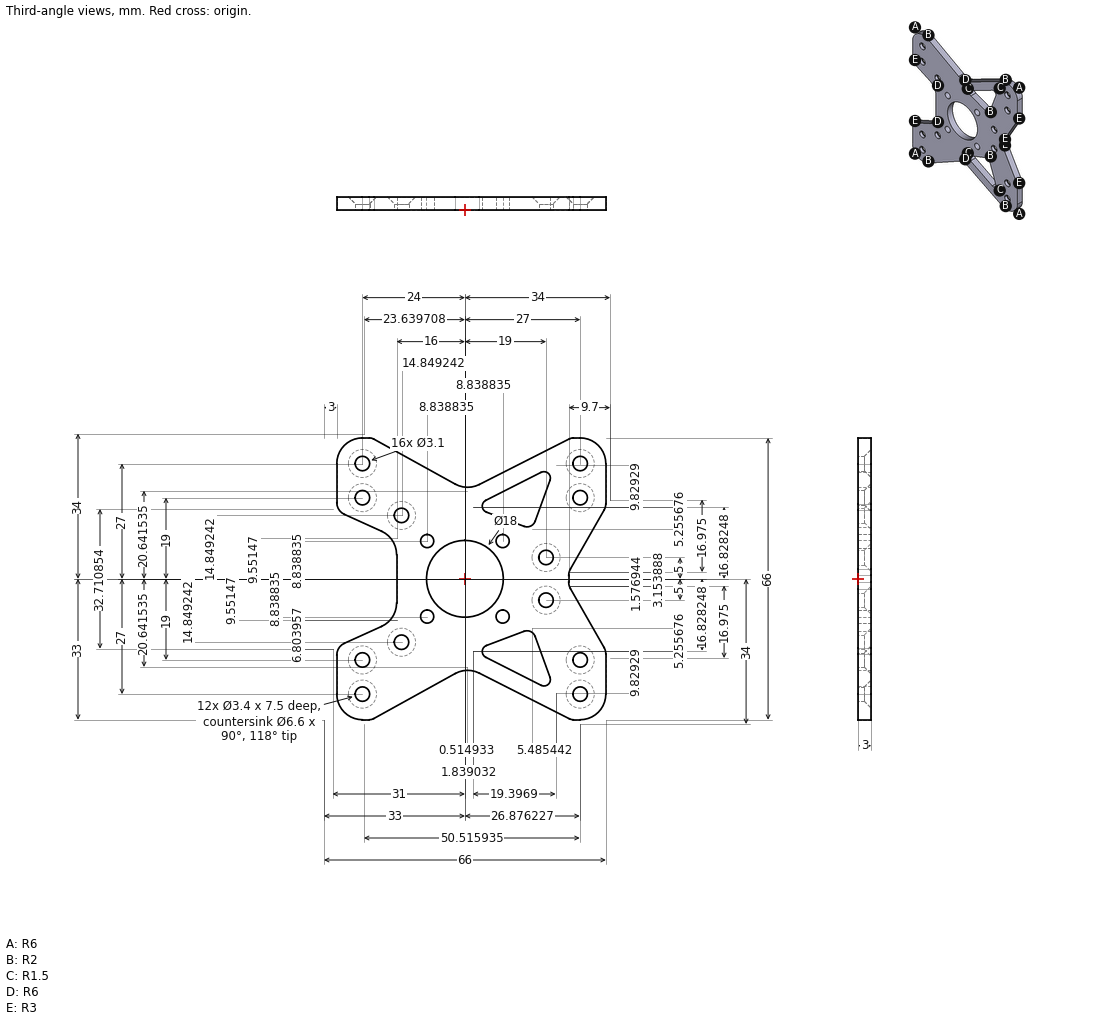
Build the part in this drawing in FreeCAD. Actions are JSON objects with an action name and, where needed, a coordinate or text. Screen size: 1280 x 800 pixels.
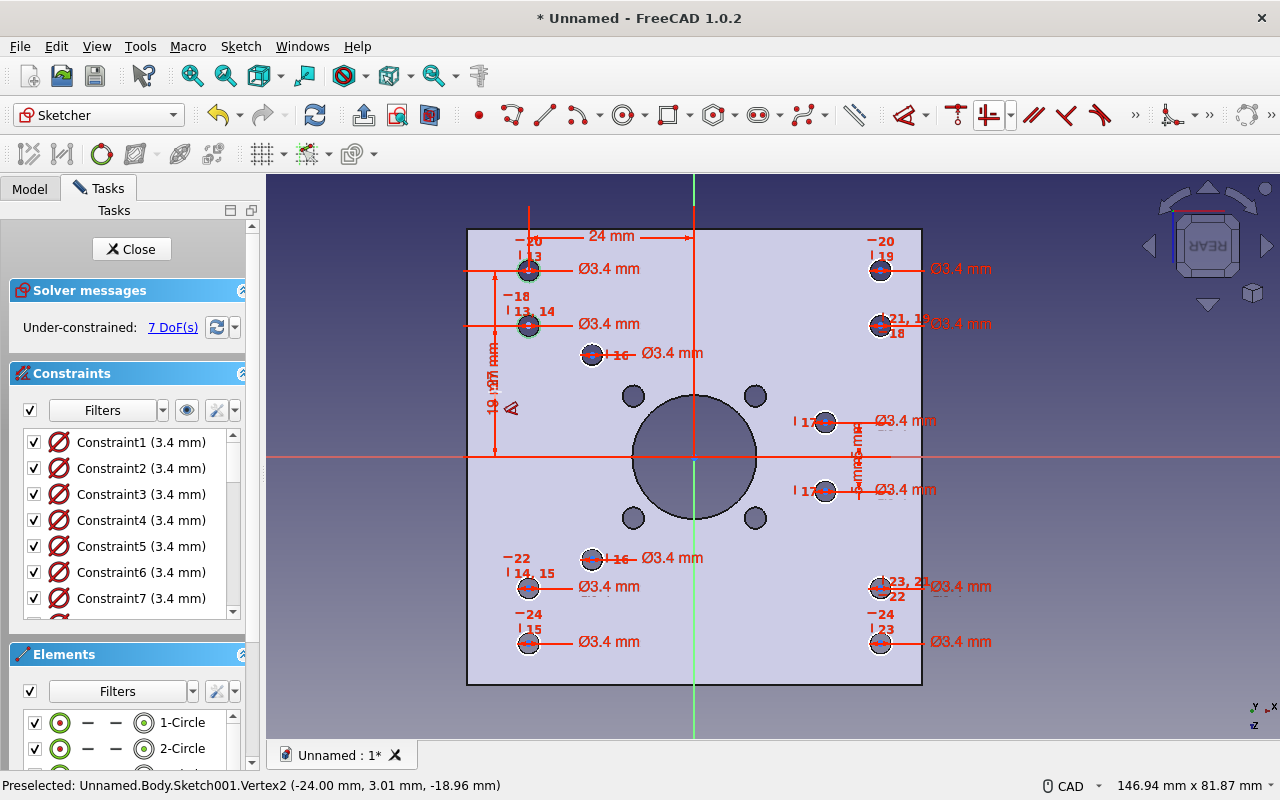
{"action": "left_click", "coordinate": [529, 589]}
{"action": "left_click", "coordinate": [495, 523]}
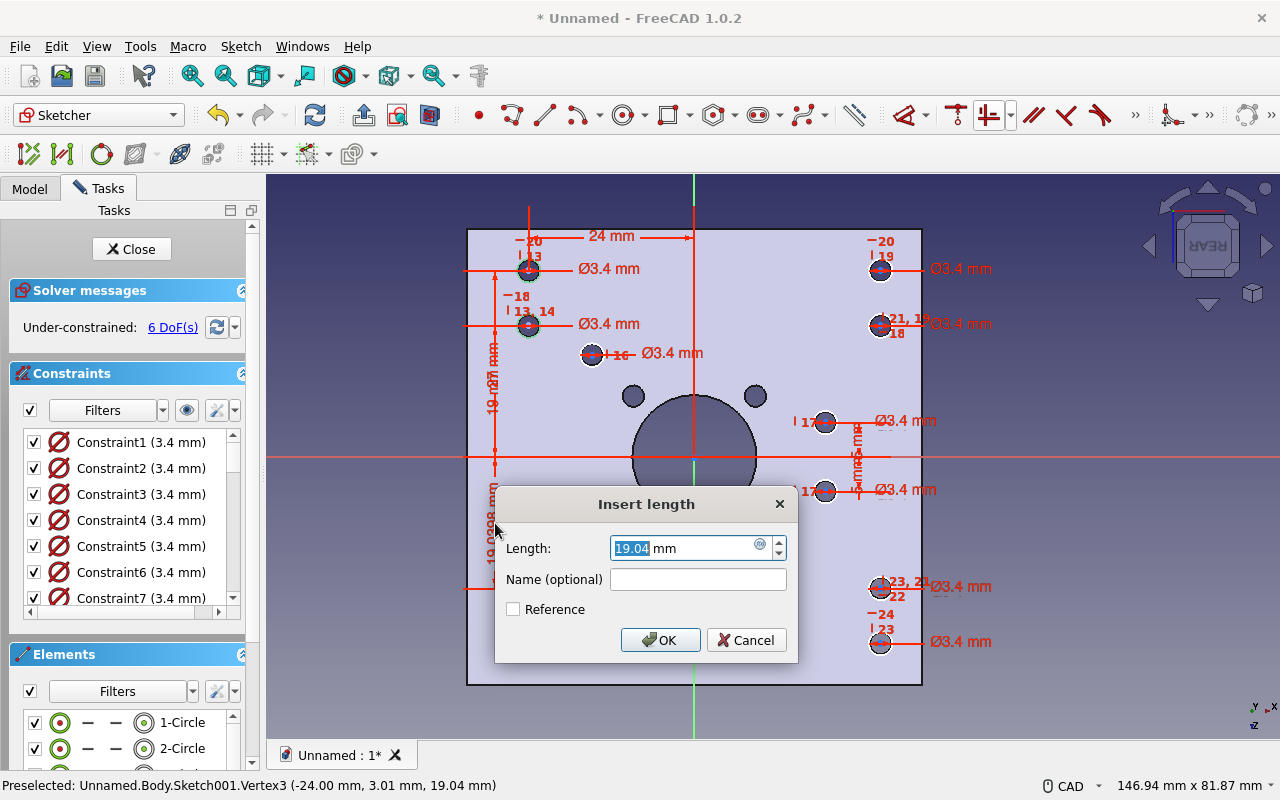
{"action": "type", "text": "19"}
{"action": "key", "text": "Return"}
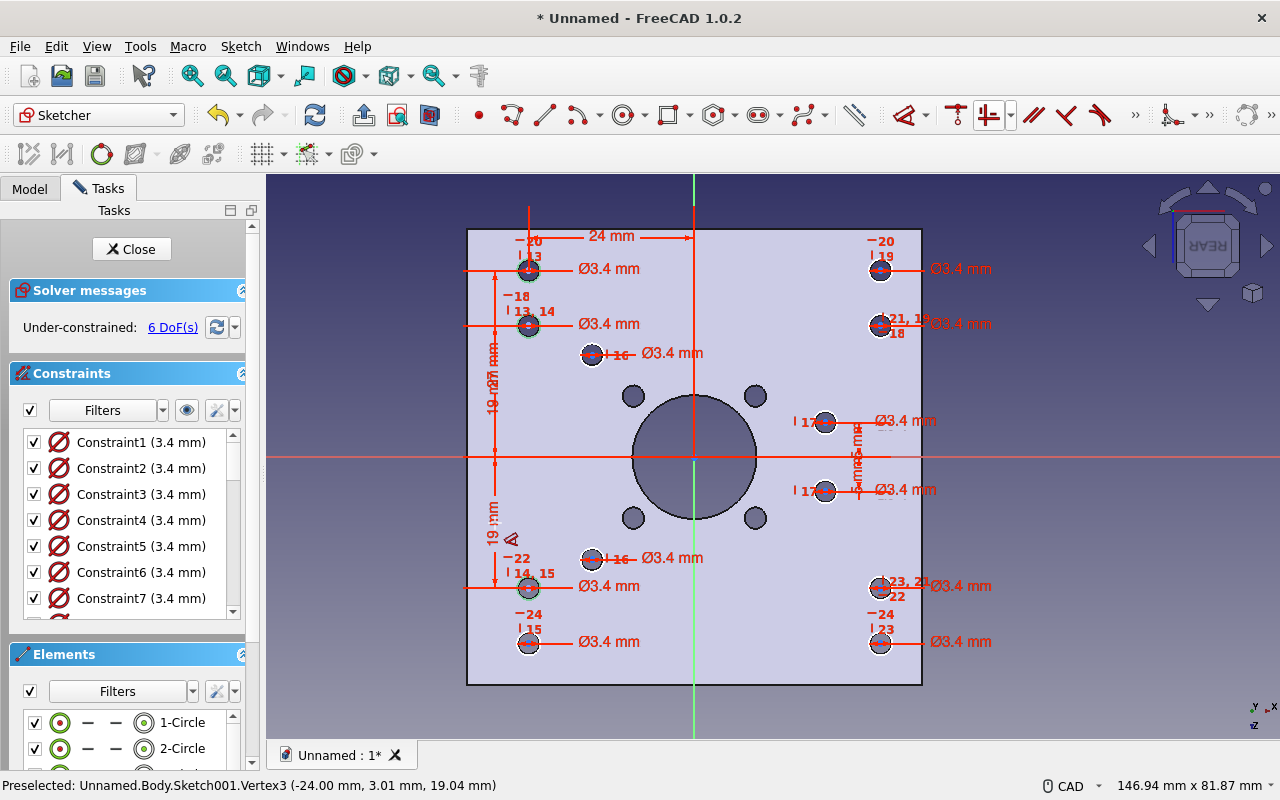
{"action": "left_click", "coordinate": [529, 644]}
{"action": "left_click", "coordinate": [495, 550]}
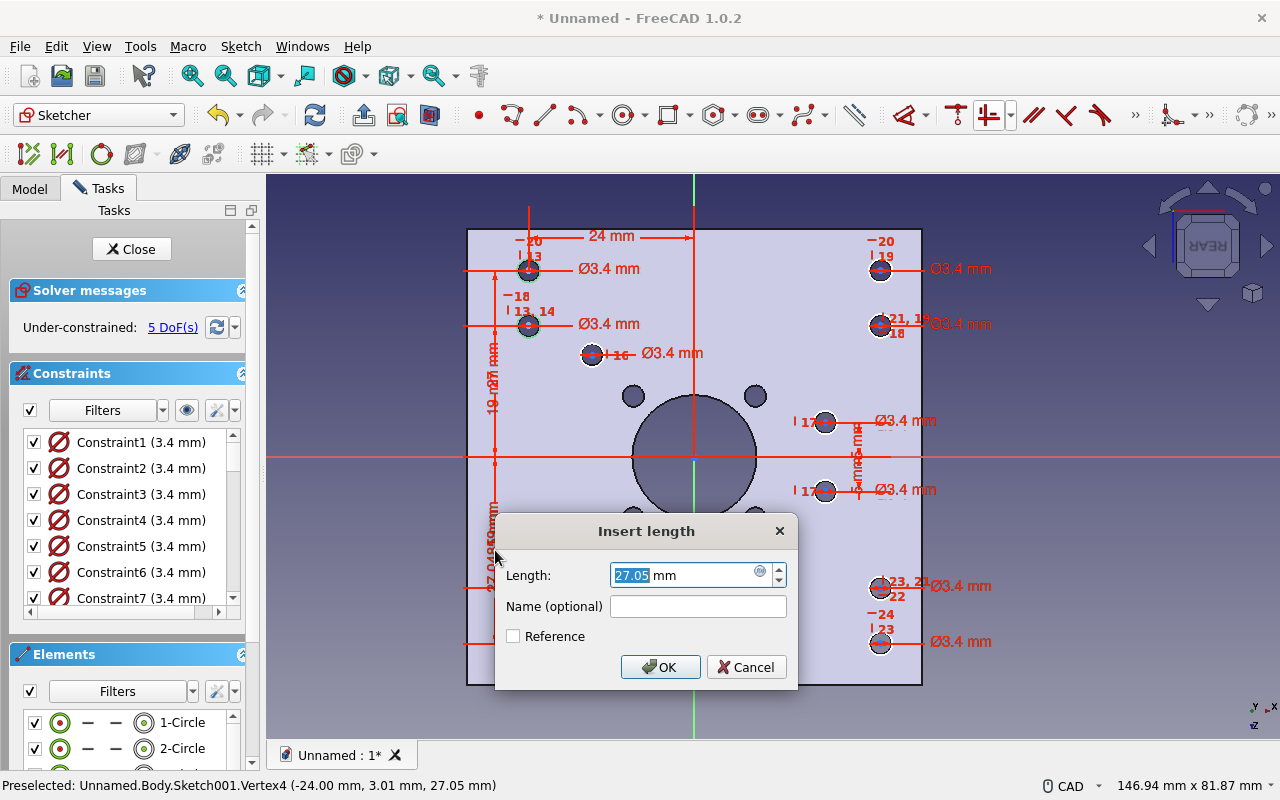
{"action": "type", "text": "27"}
{"action": "key", "text": "Return"}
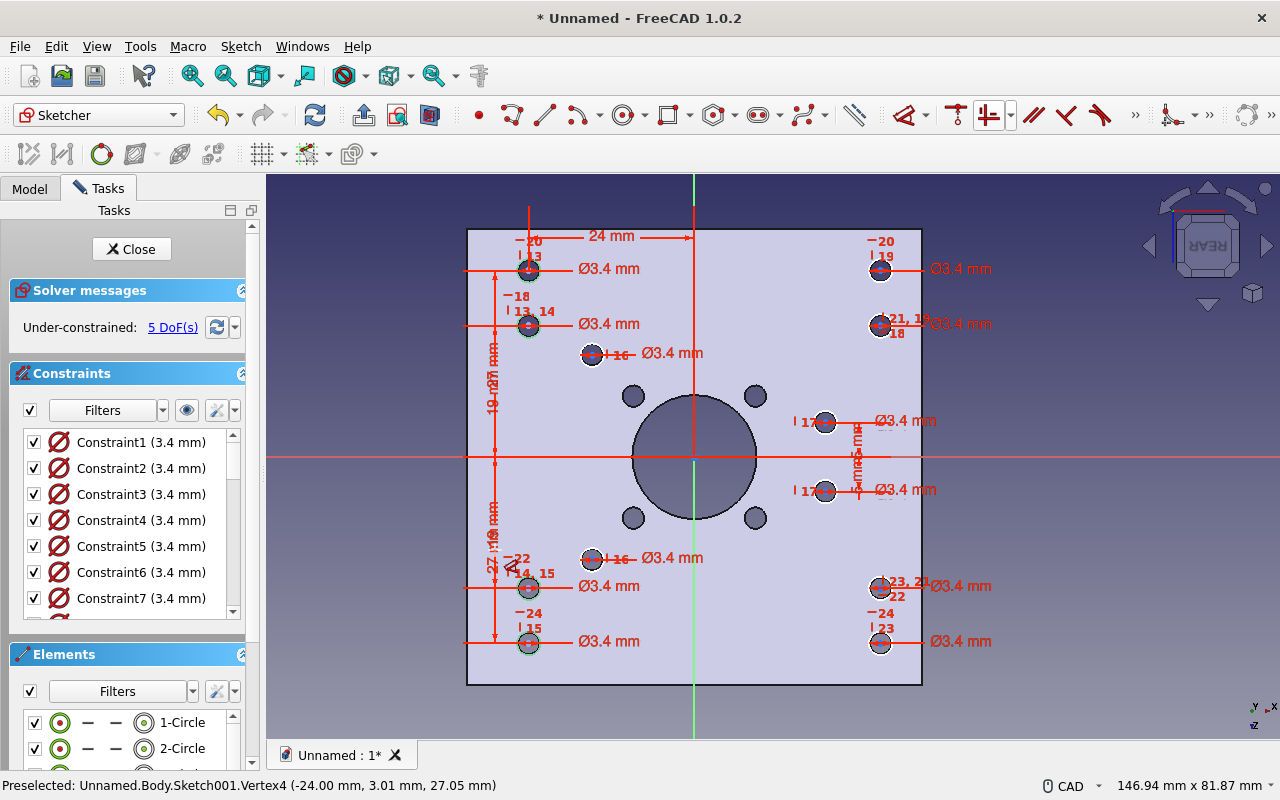
{"action": "left_click", "coordinate": [825, 492]}
{"action": "left_click", "coordinate": [760, 526]}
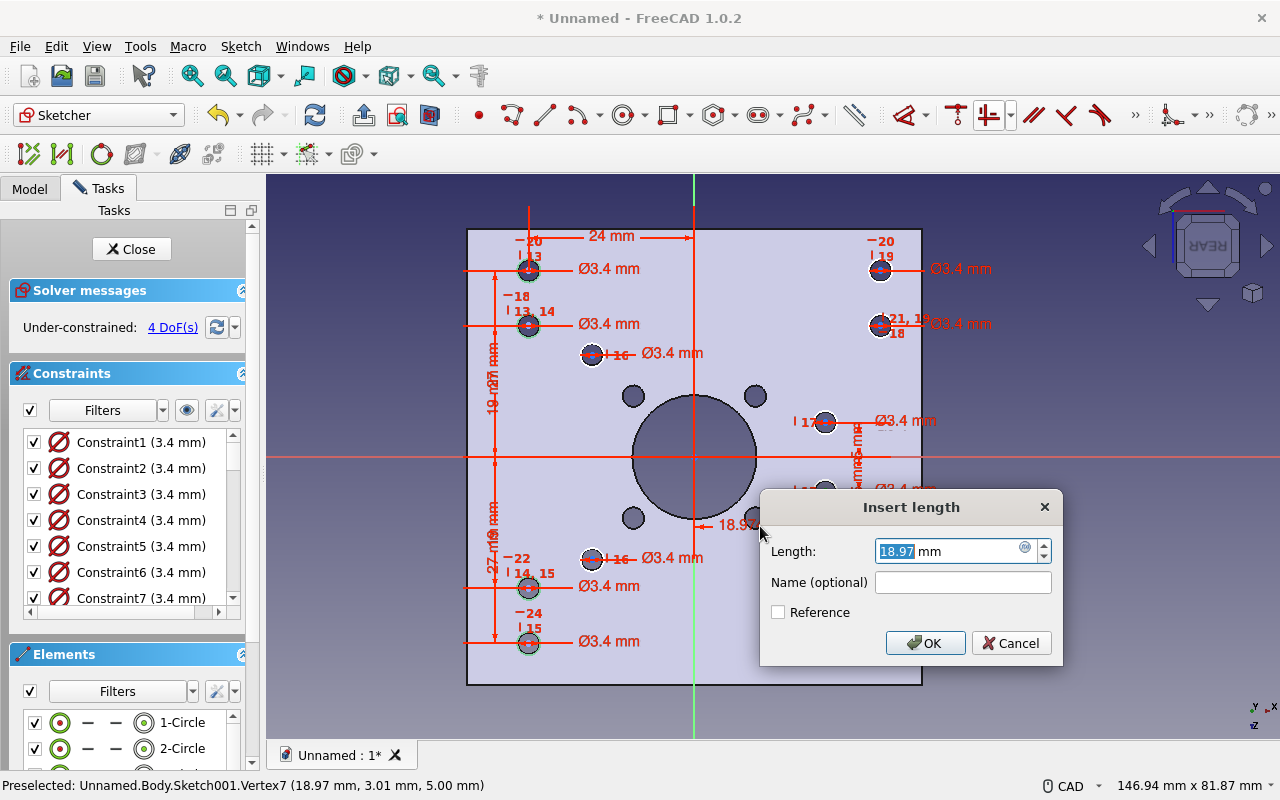
{"action": "type", "text": "19"}
{"action": "key", "text": "Return"}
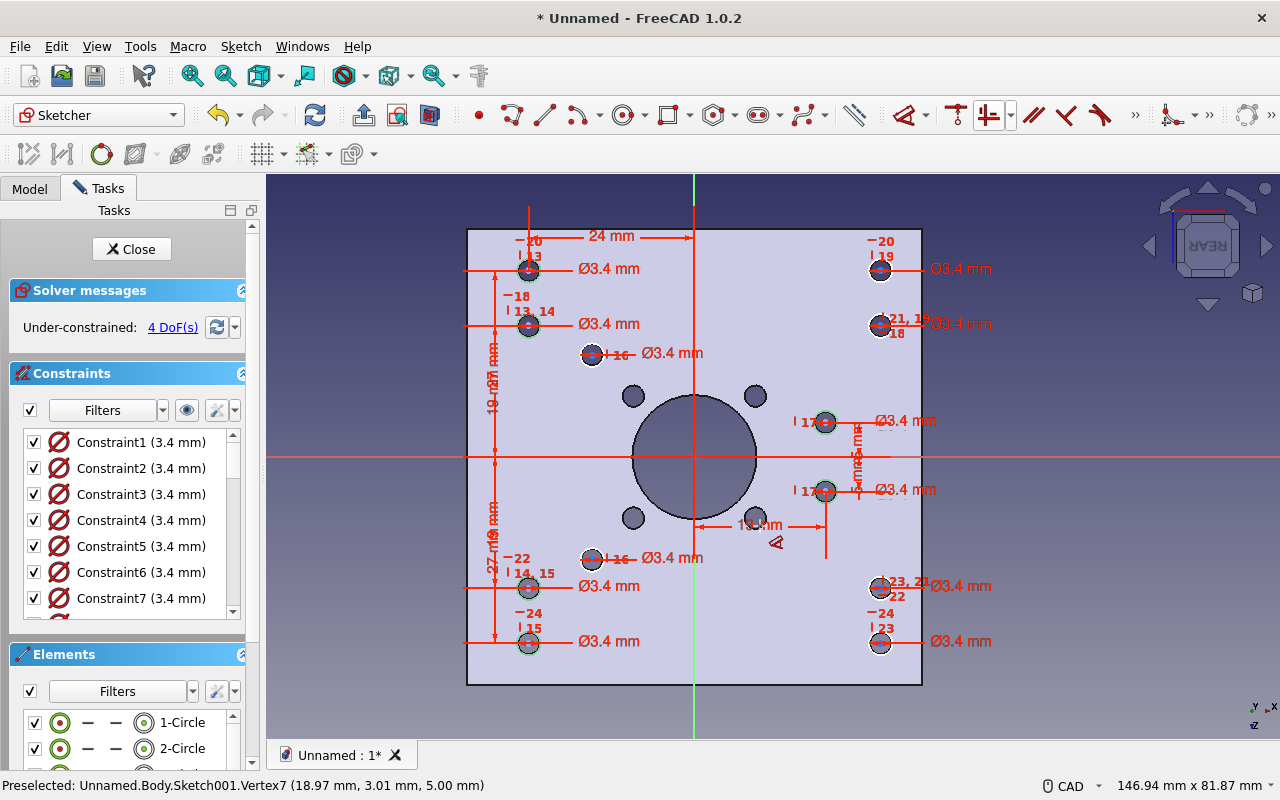
{"action": "left_click", "coordinate": [881, 326]}
{"action": "left_click", "coordinate": [788, 292]}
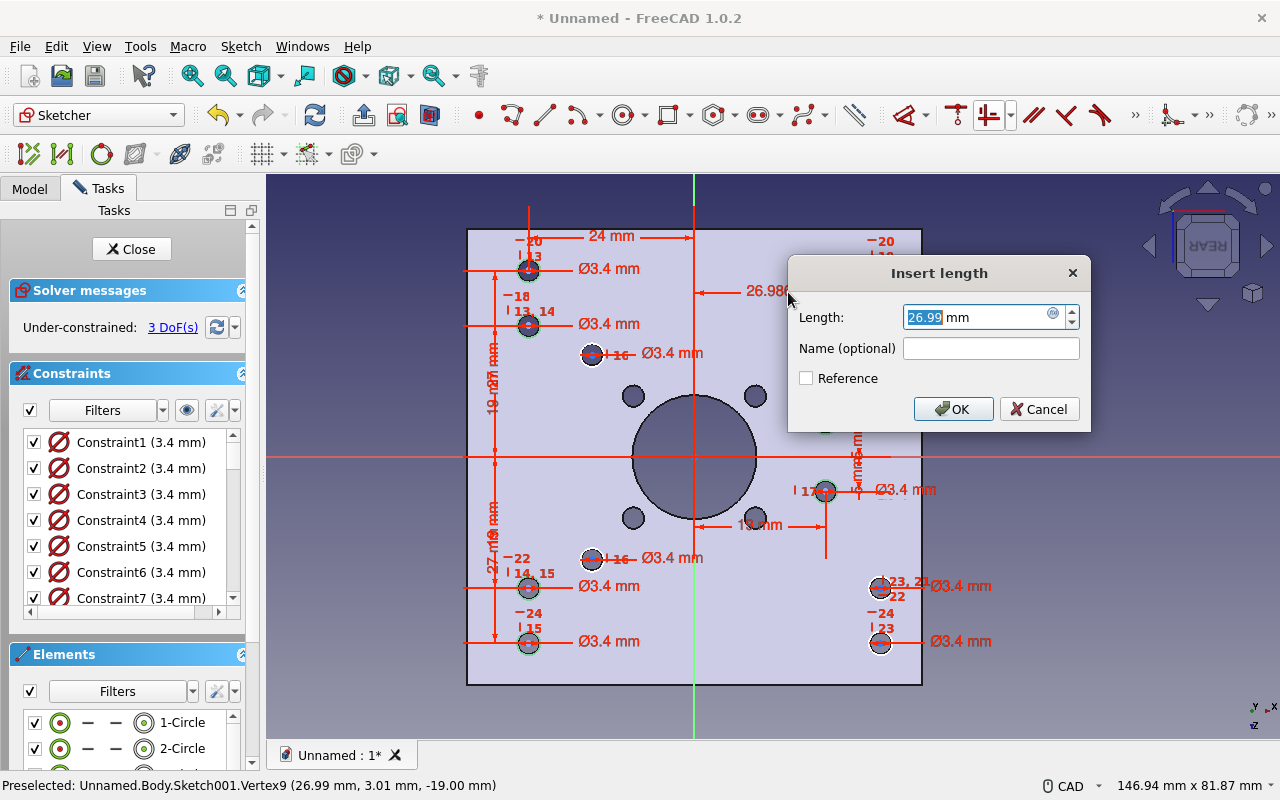
{"action": "type", "text": "27"}
{"action": "key", "text": "Return"}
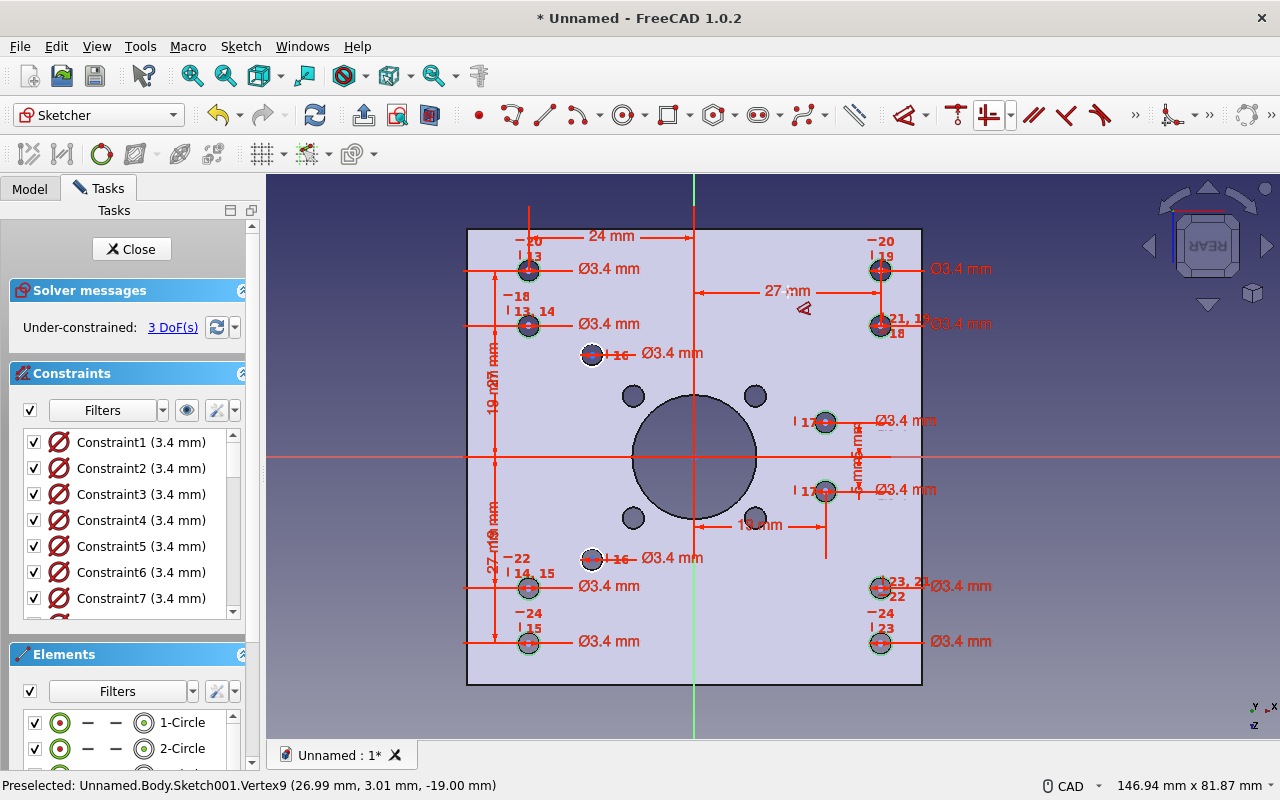
{"action": "left_click", "coordinate": [592, 355]}
{"action": "left_click", "coordinate": [643, 321]}